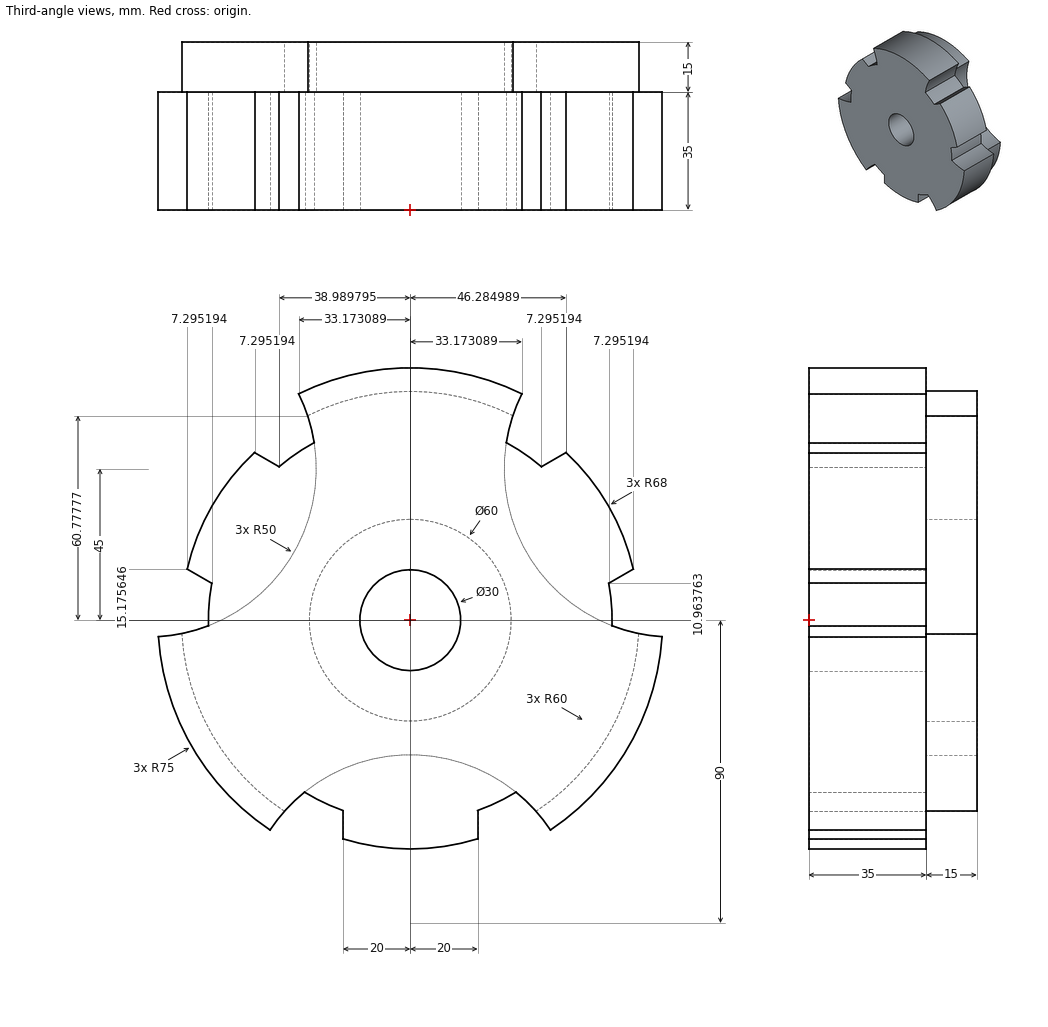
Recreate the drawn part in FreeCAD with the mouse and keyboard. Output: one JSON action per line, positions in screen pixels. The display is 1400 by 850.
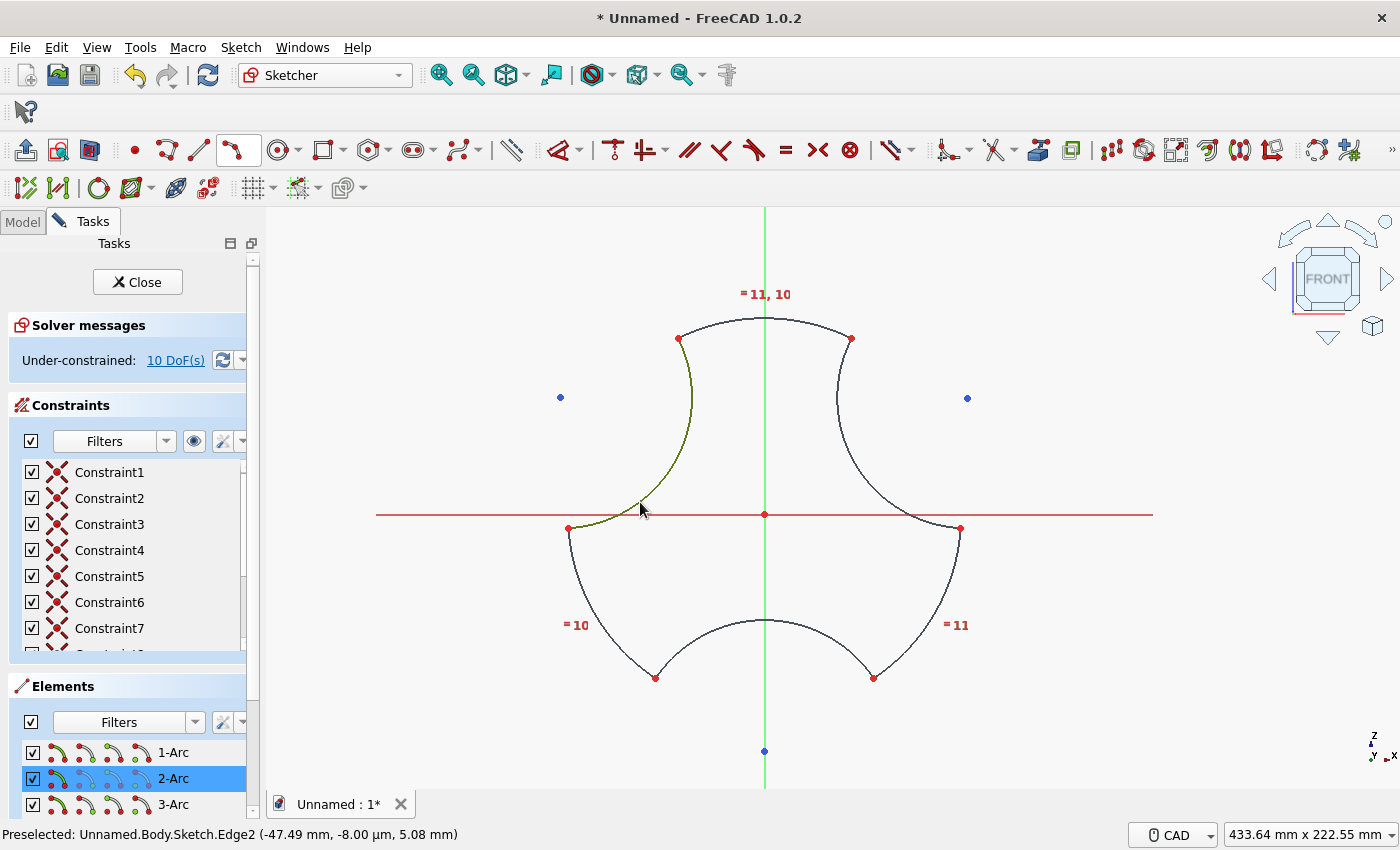
{"action": "left_click", "coordinate": [838, 414]}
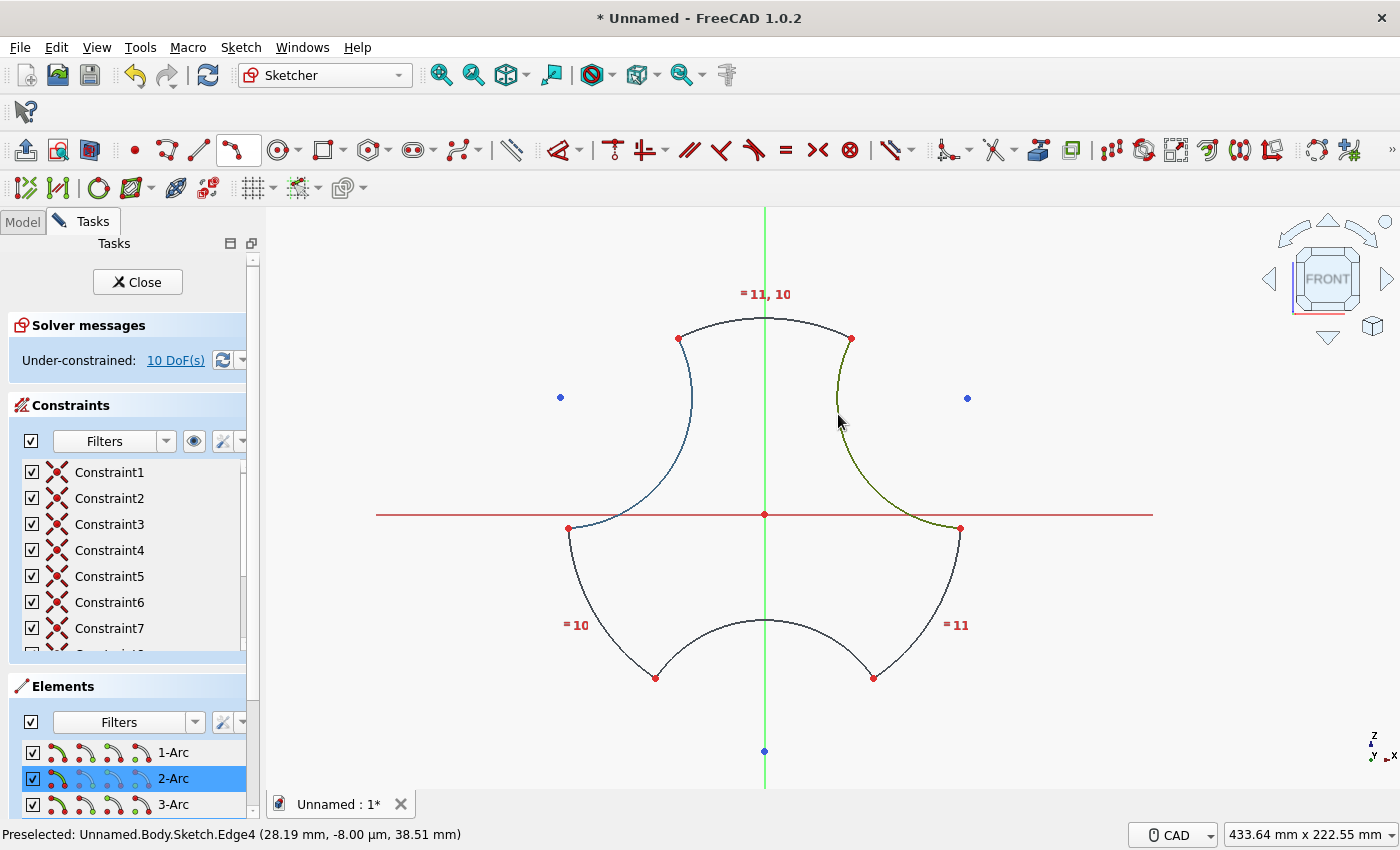
{"action": "left_click", "coordinate": [815, 630]}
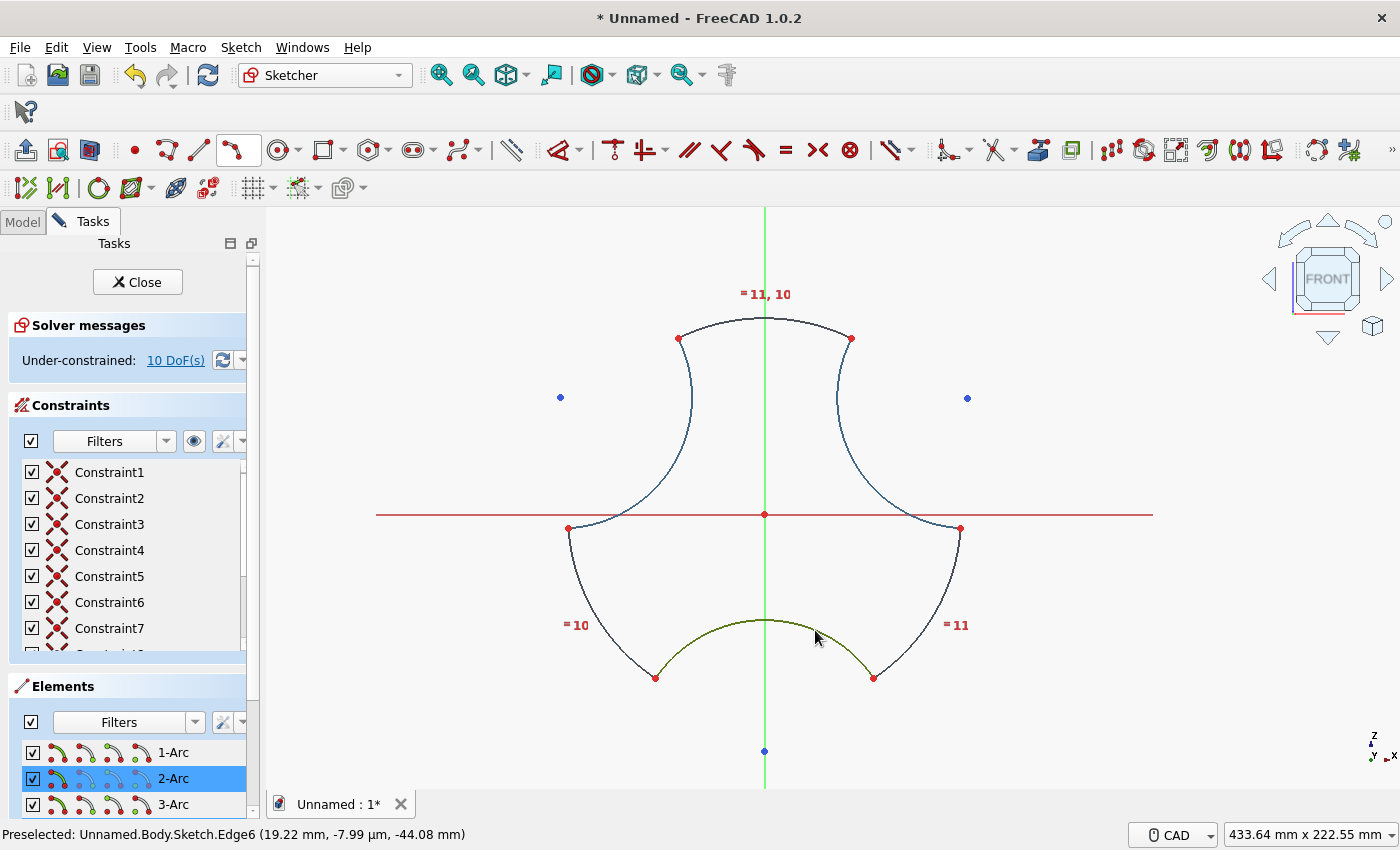
{"action": "left_click", "coordinate": [786, 150]}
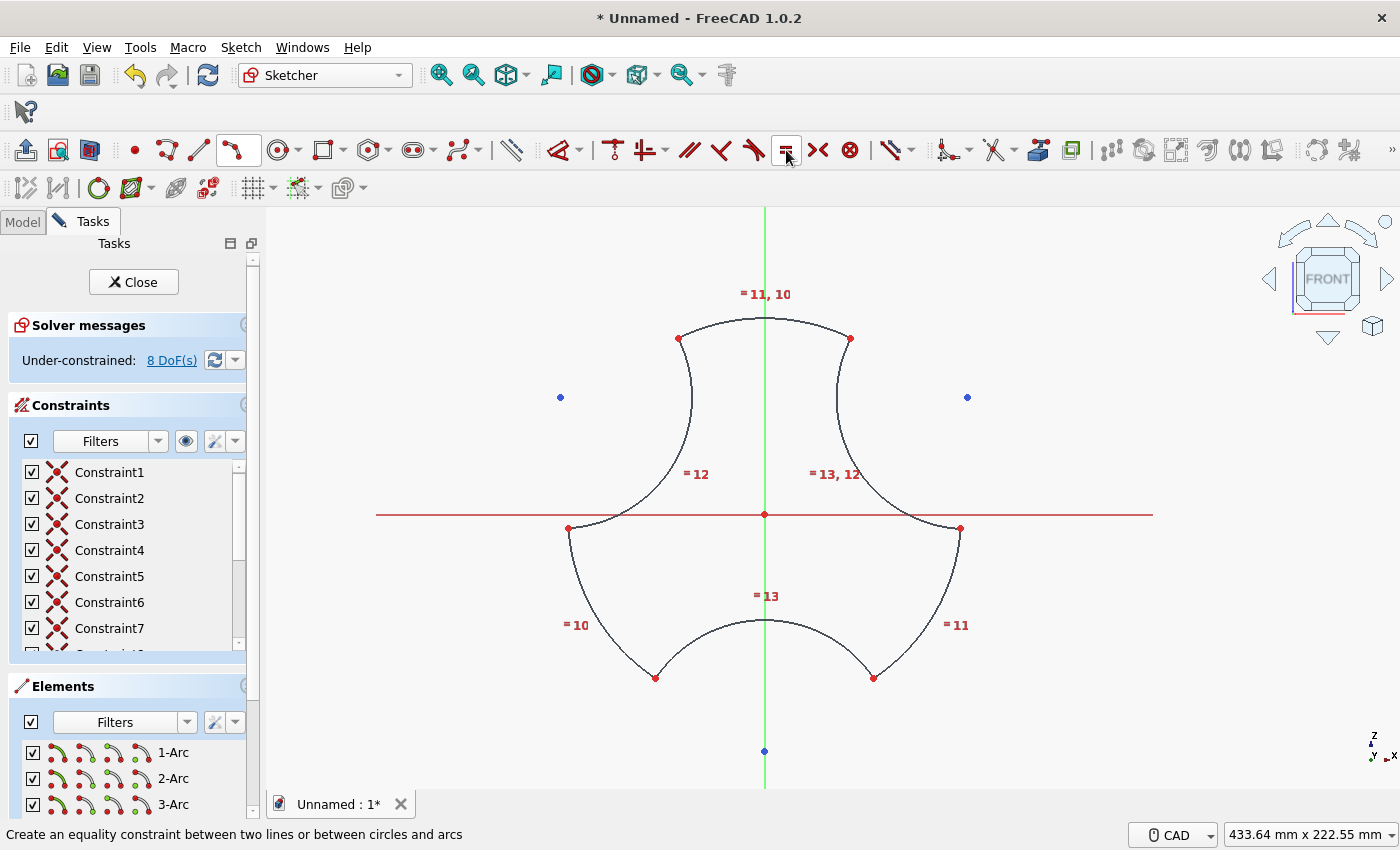
{"action": "left_click", "coordinate": [765, 751]}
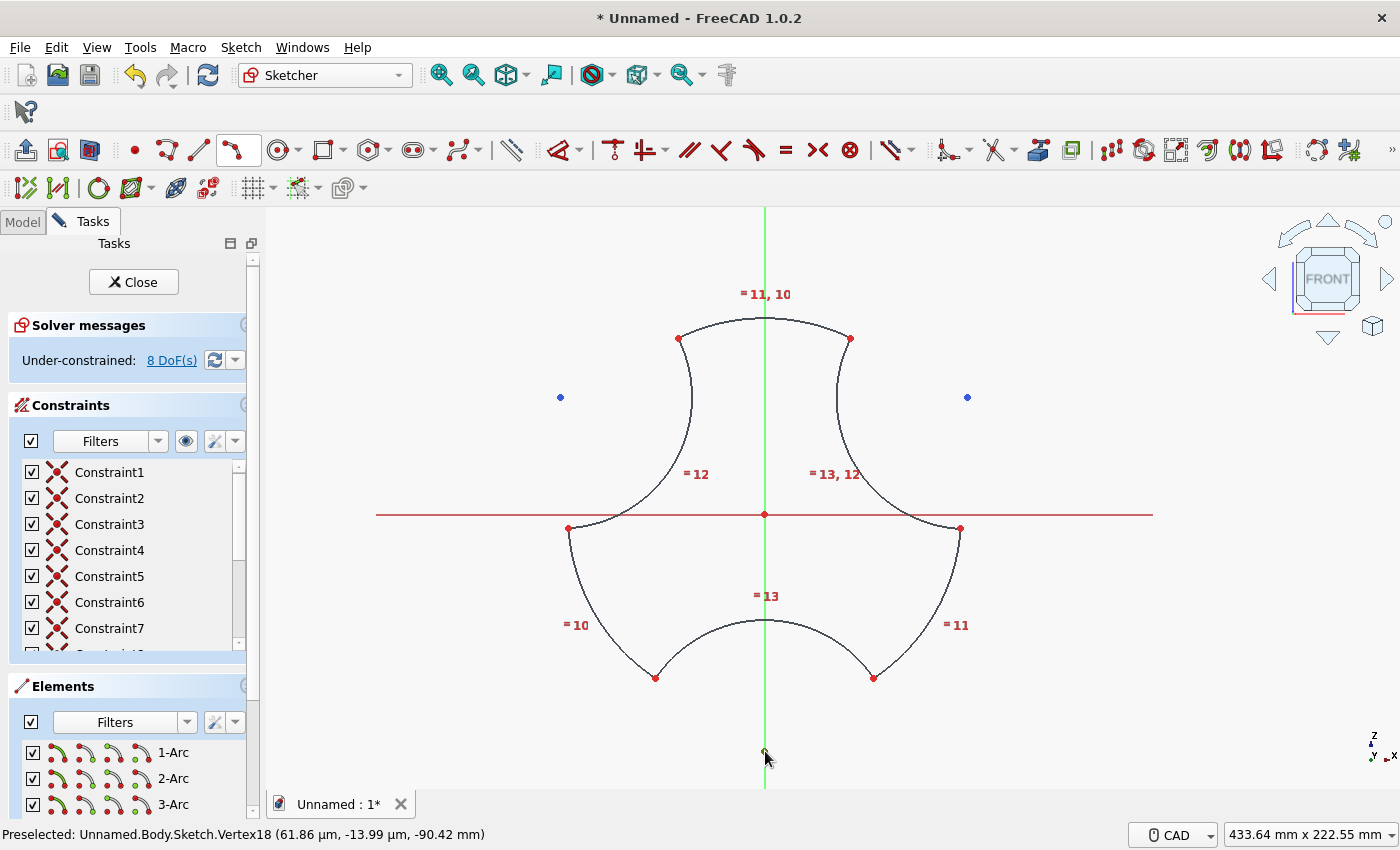
{"action": "left_click", "coordinate": [765, 723]}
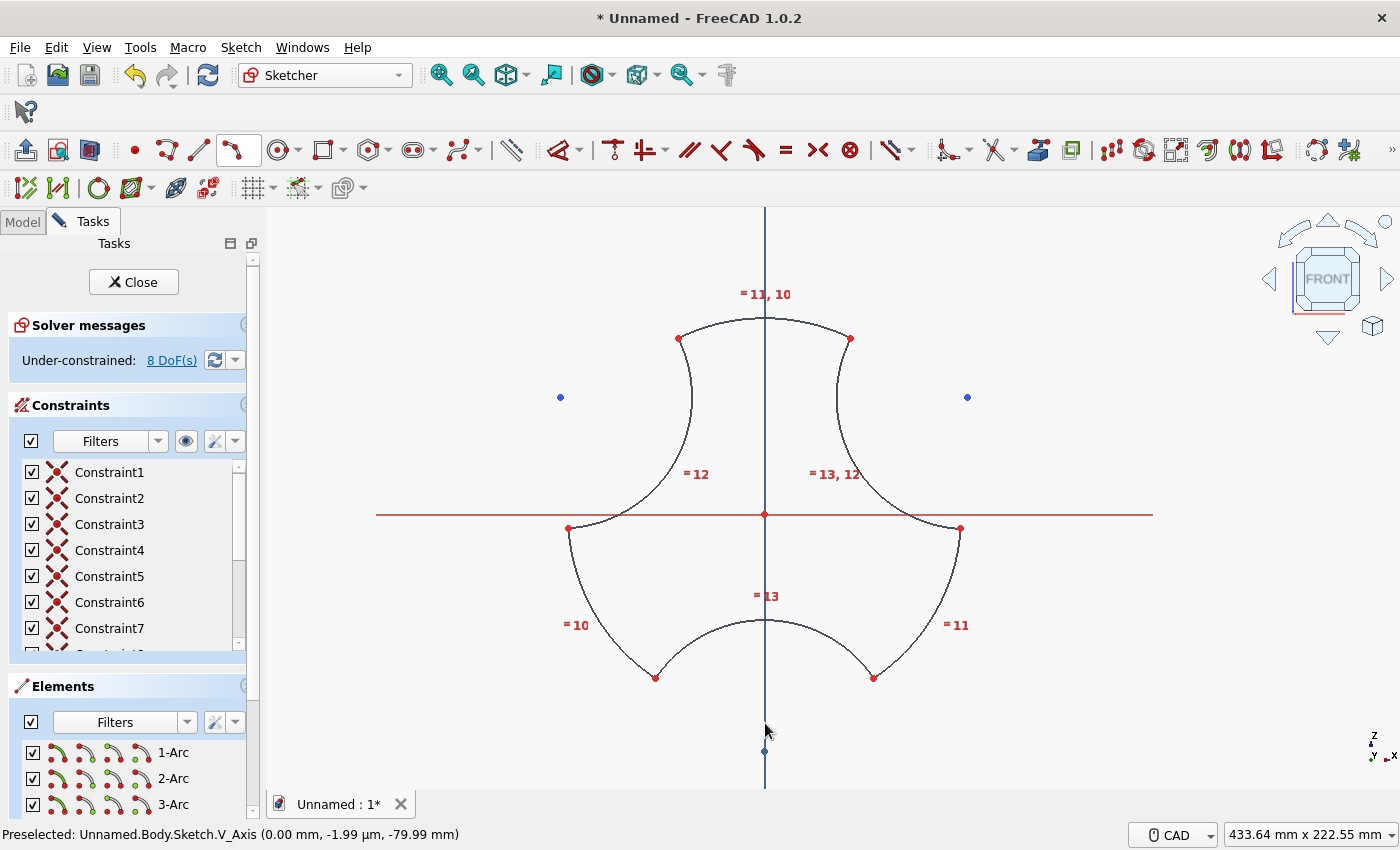
{"action": "left_click", "coordinate": [614, 150]}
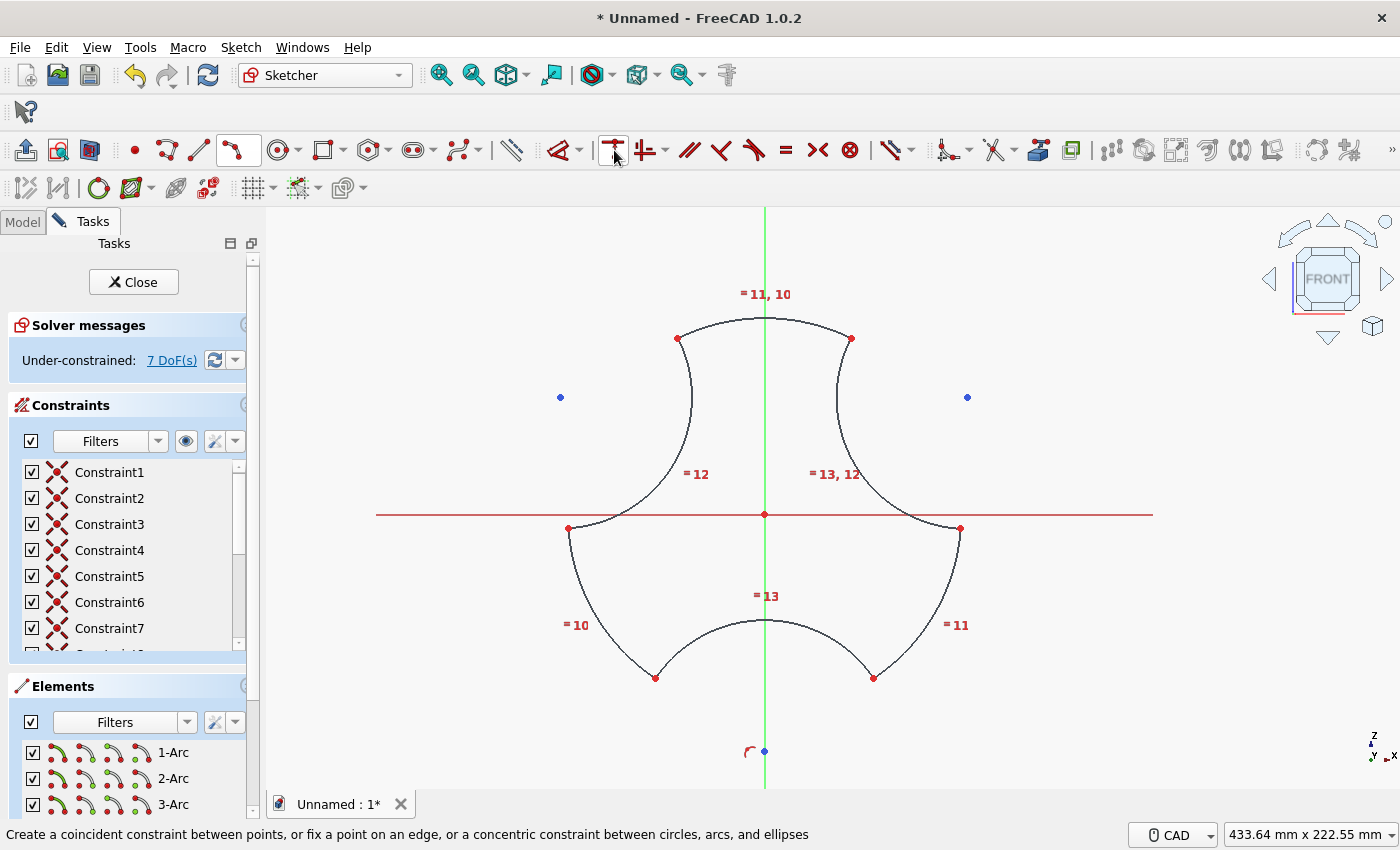
{"action": "left_click", "coordinate": [558, 150]}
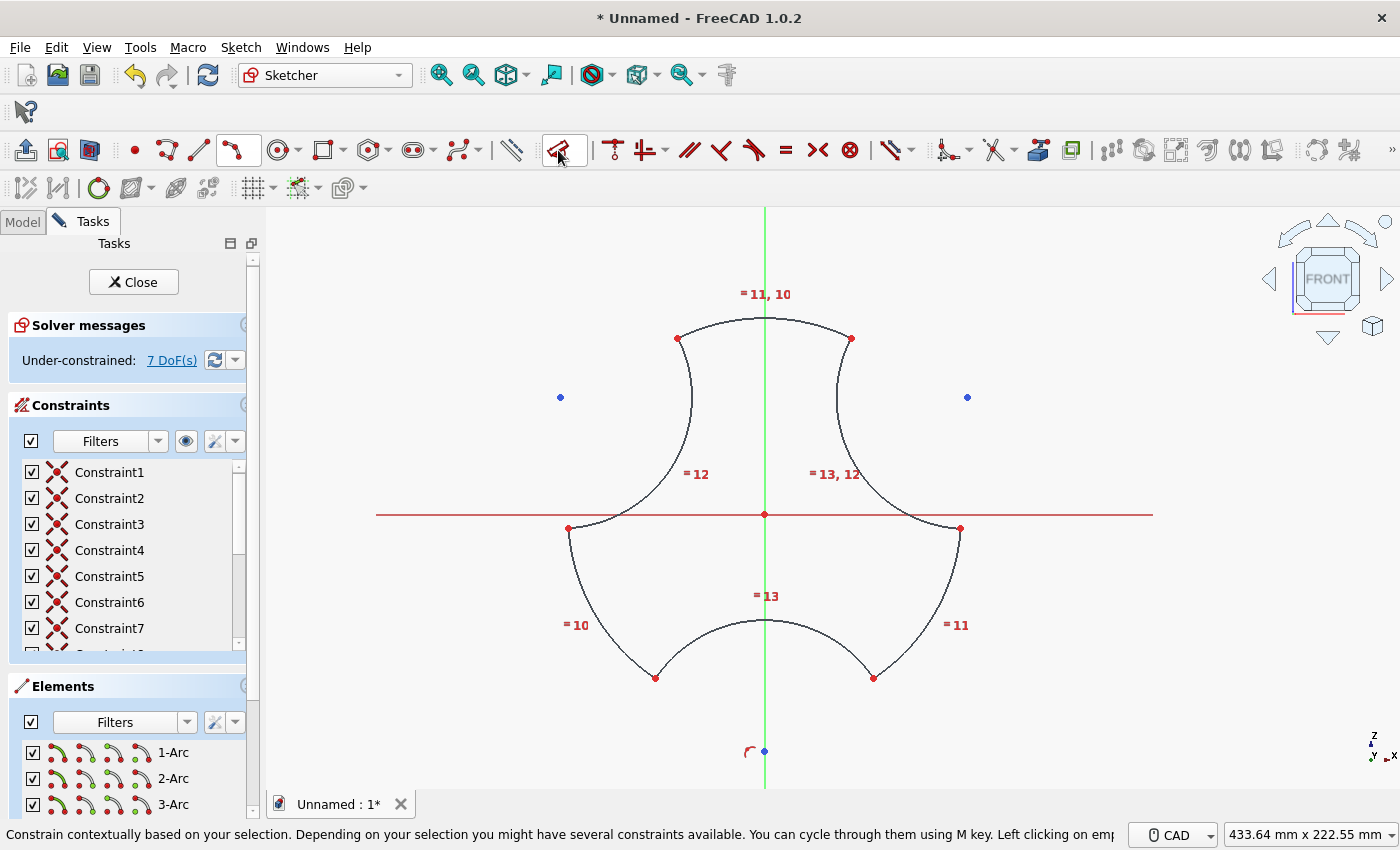
{"action": "left_click", "coordinate": [579, 581]}
{"action": "left_click", "coordinate": [549, 592]}